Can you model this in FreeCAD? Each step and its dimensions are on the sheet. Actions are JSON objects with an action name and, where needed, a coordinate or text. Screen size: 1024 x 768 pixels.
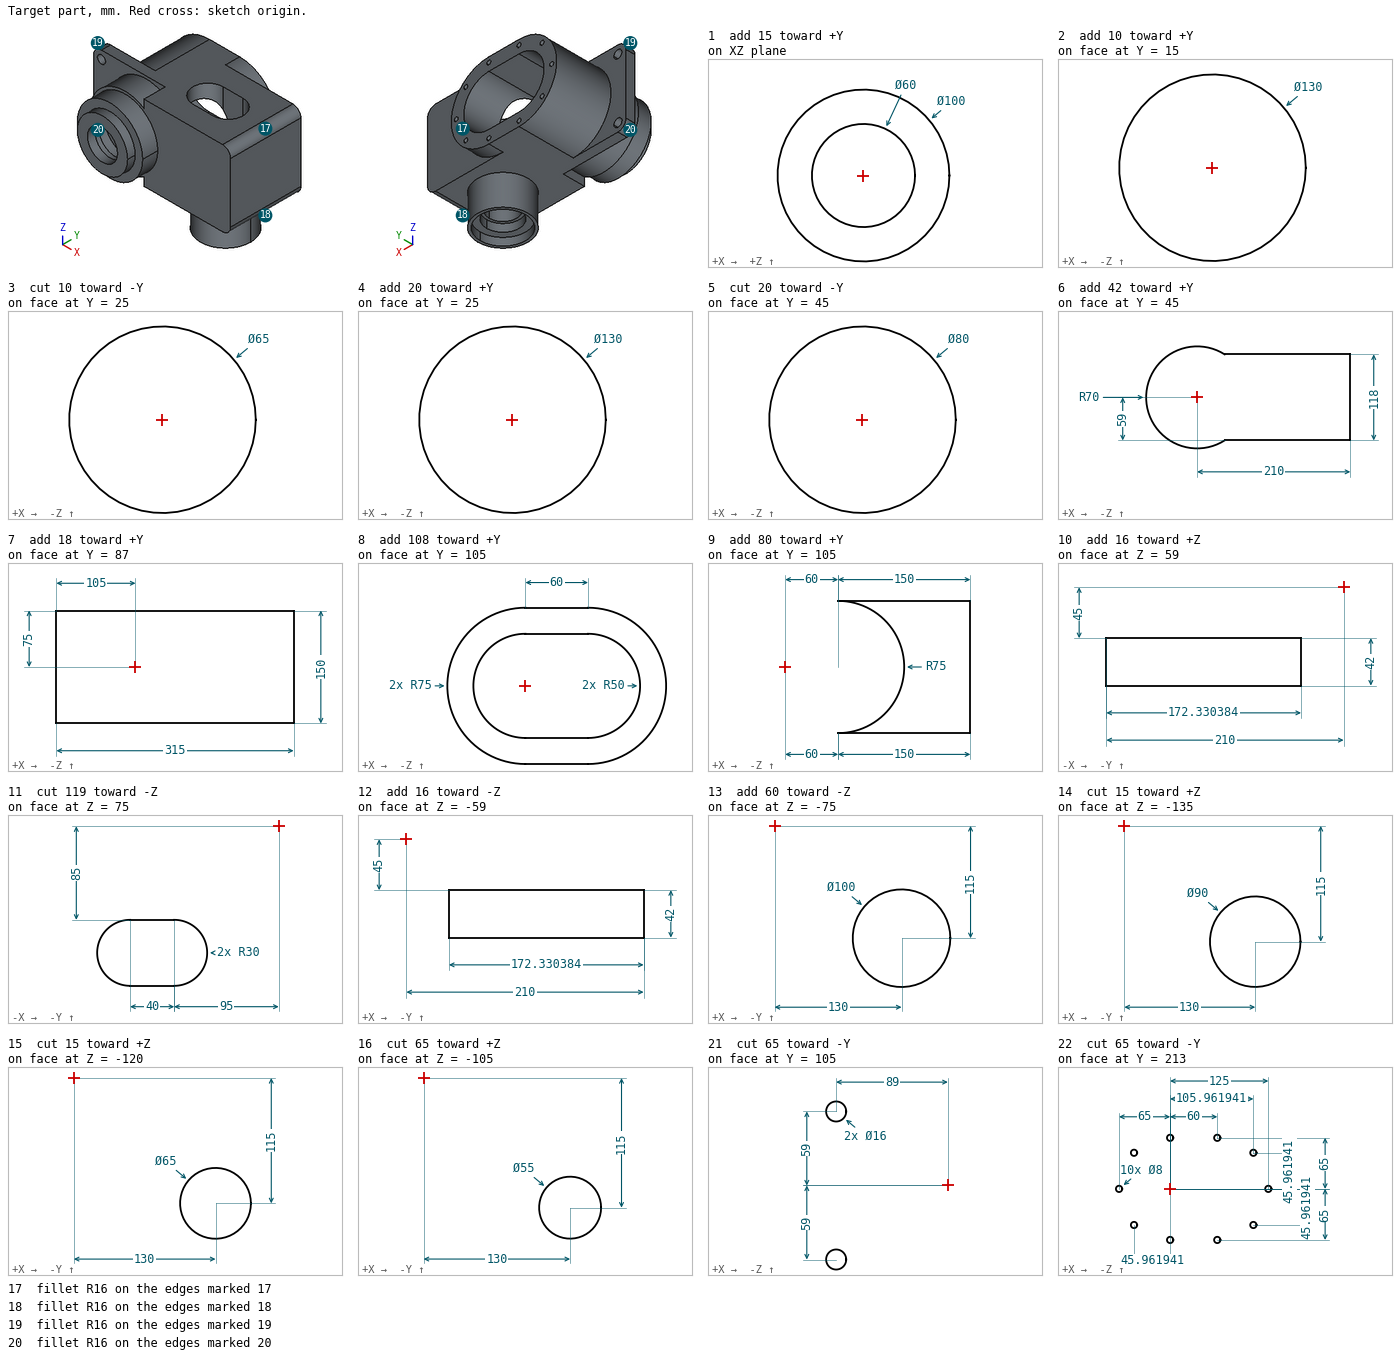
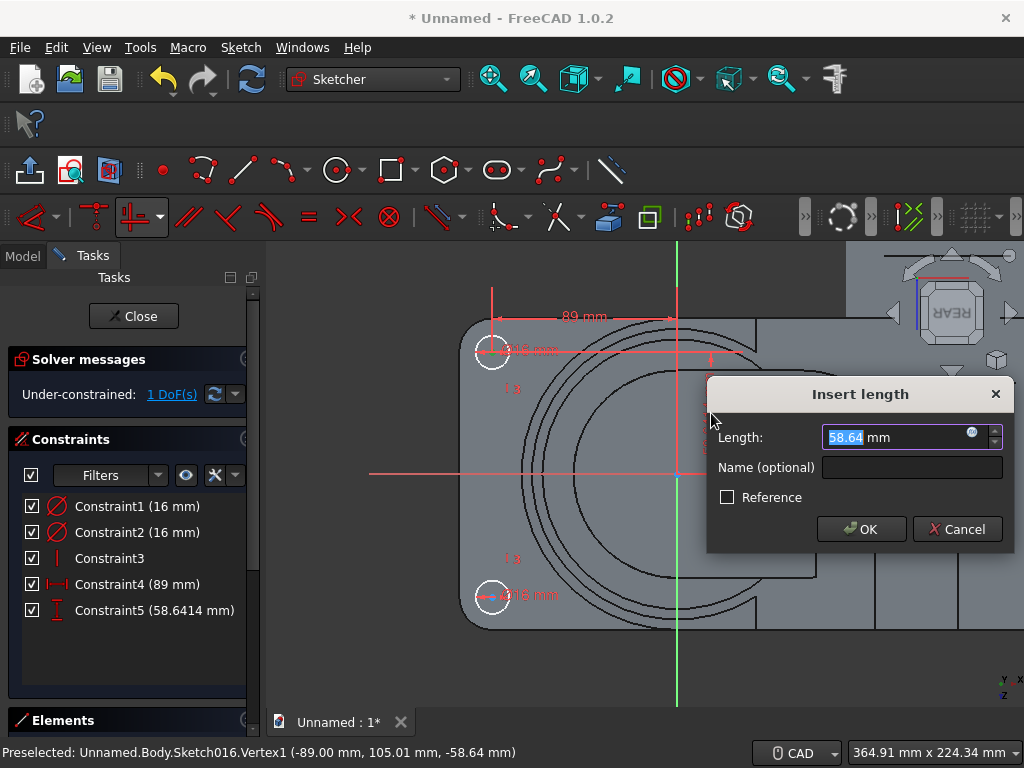
{"action": "type", "text": "59"}
{"action": "key", "text": "Return"}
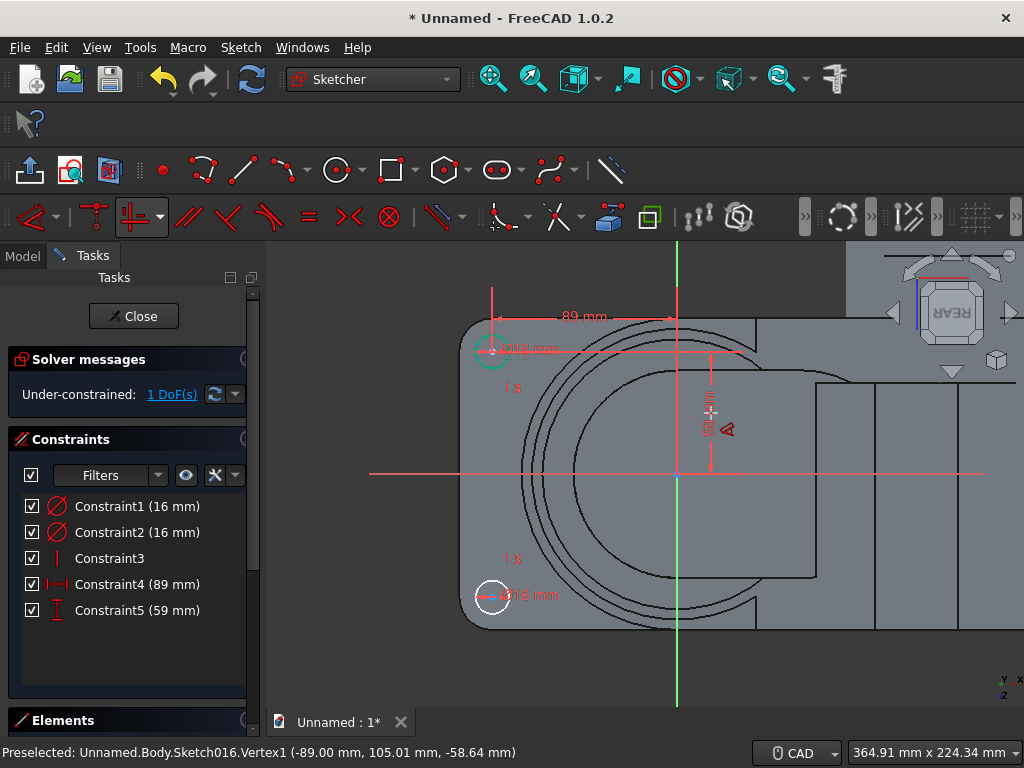
{"action": "left_click", "coordinate": [492, 597]}
{"action": "left_click", "coordinate": [711, 536]}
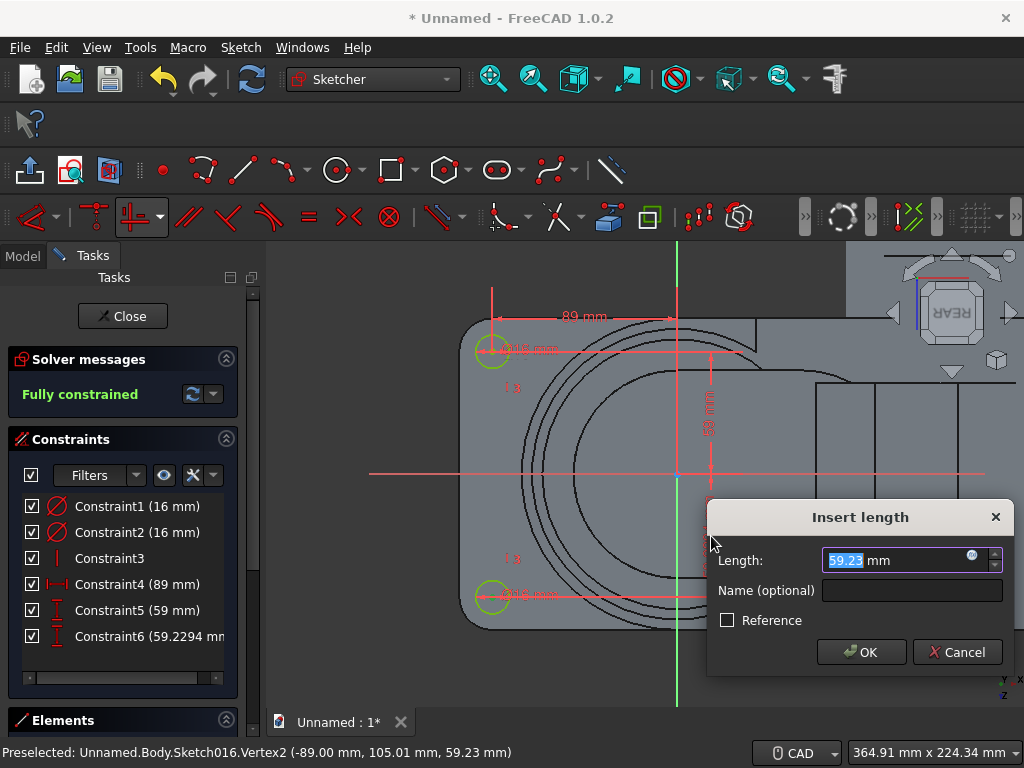
{"action": "type", "text": "59"}
{"action": "key", "text": "Return"}
{"action": "key", "text": "Escape"}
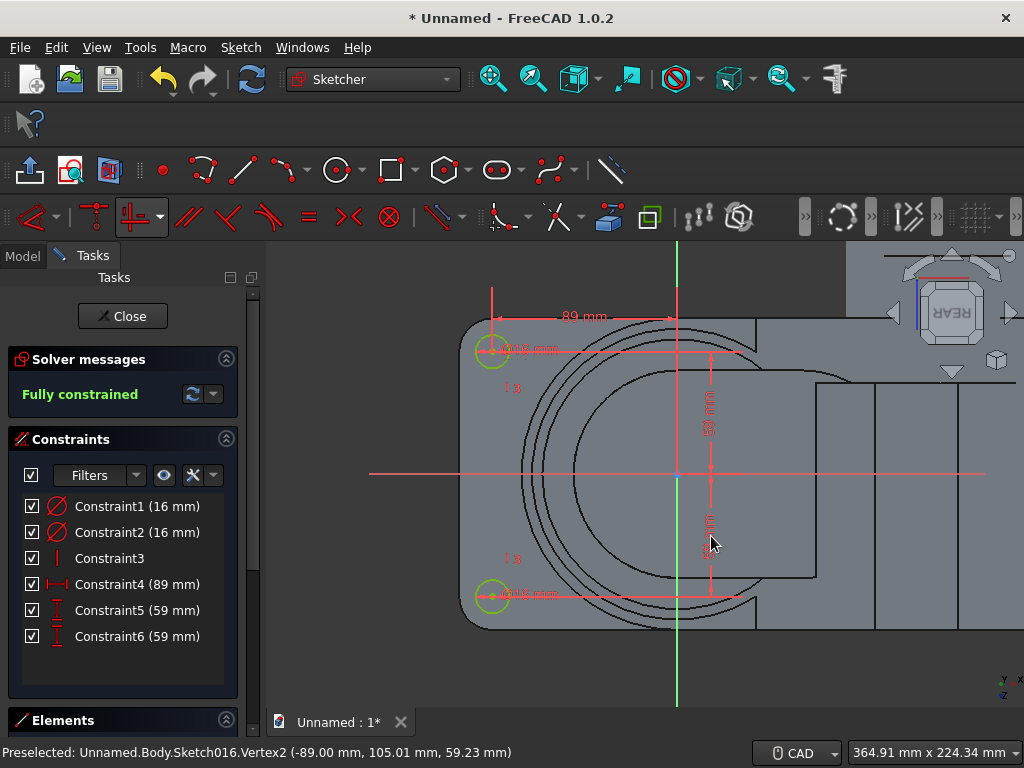
{"action": "left_click", "coordinate": [123, 316]}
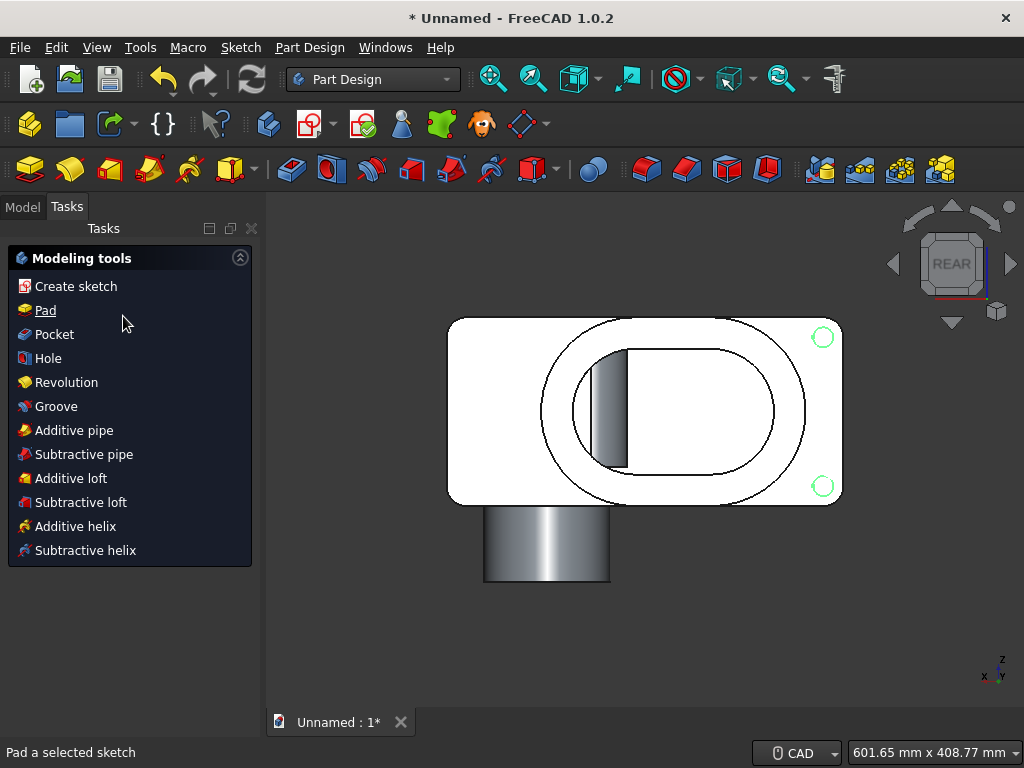
{"action": "left_click", "coordinate": [292, 170]}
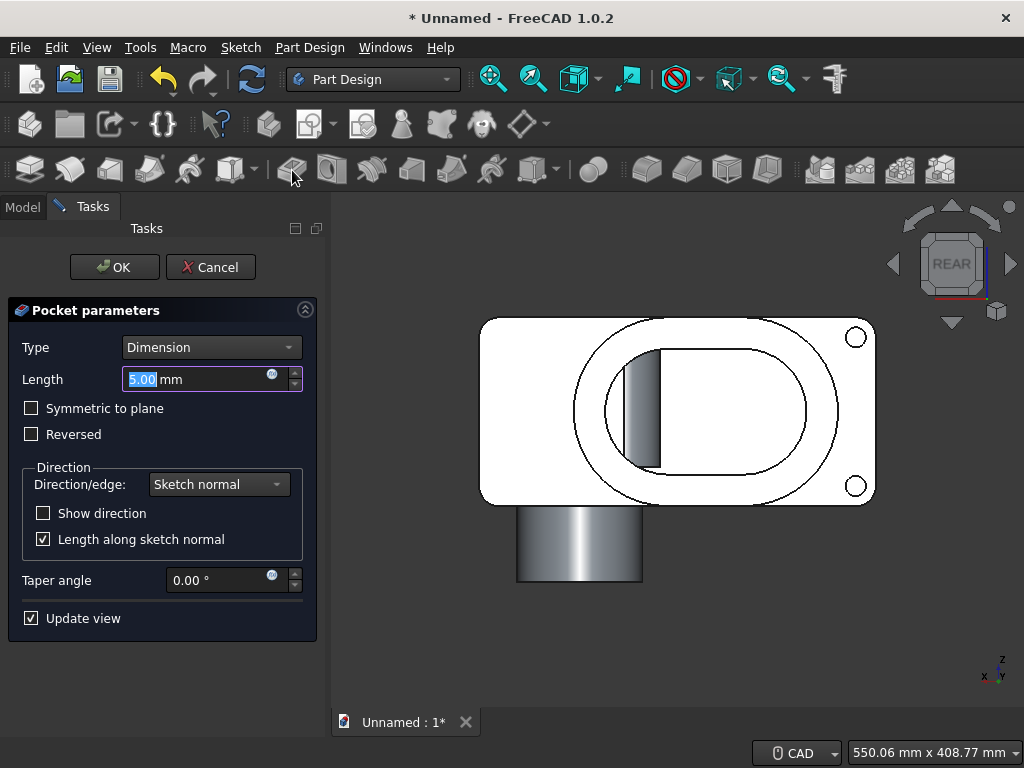
{"action": "type", "text": "65"}
{"action": "key", "text": "Tab"}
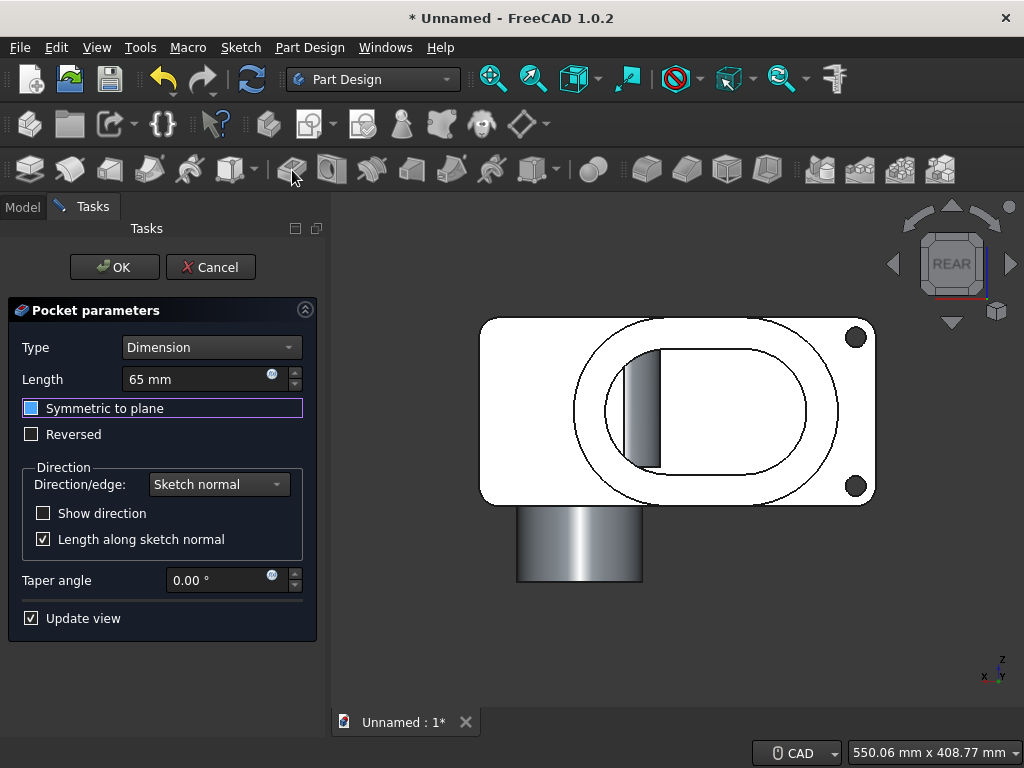
{"action": "left_click", "coordinate": [115, 267]}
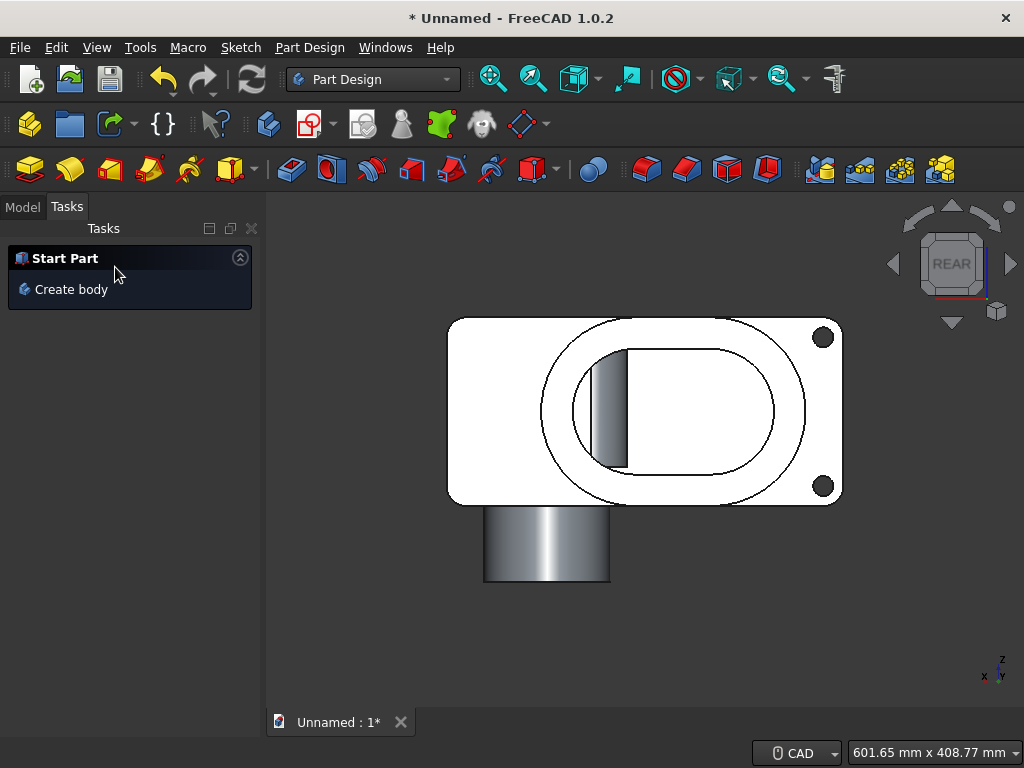
{"action": "left_click", "coordinate": [560, 438]}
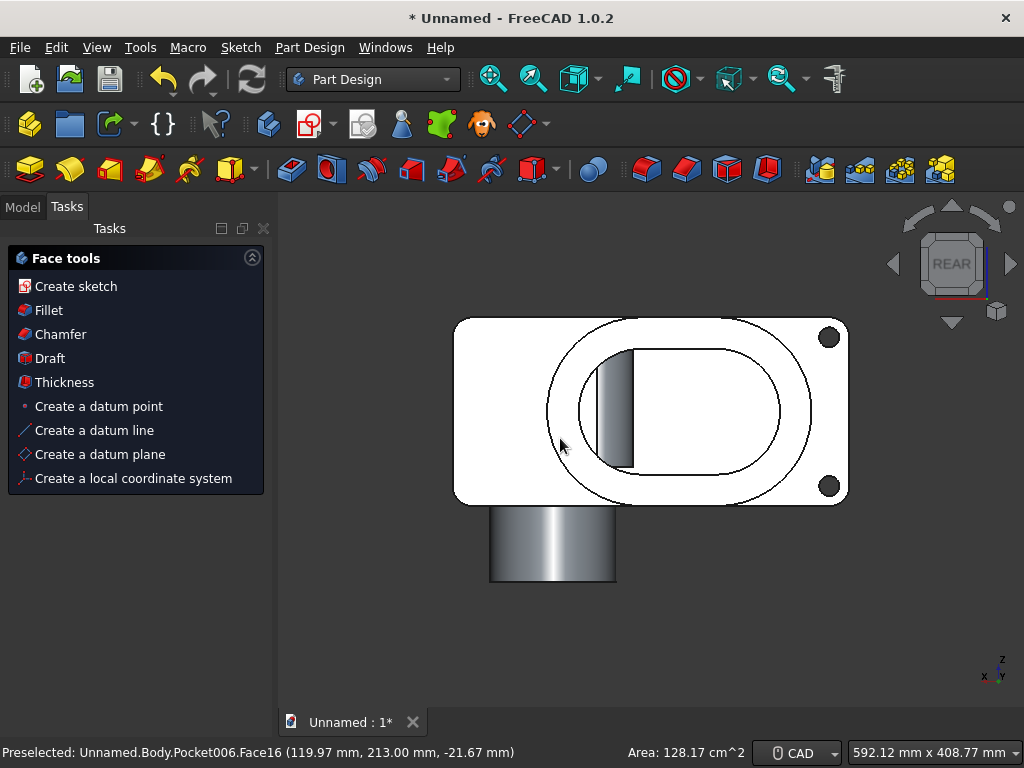
{"action": "left_click", "coordinate": [310, 124]}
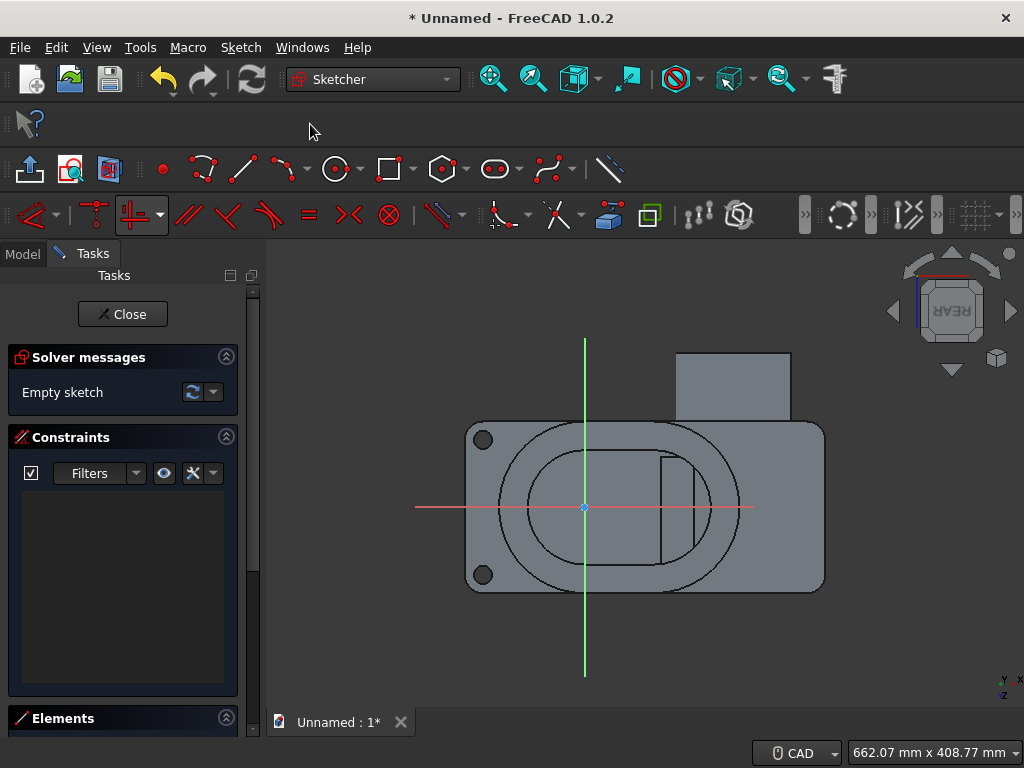
{"action": "scroll", "coordinate": [671, 549], "scroll_direction": "up", "scroll_amount": 3}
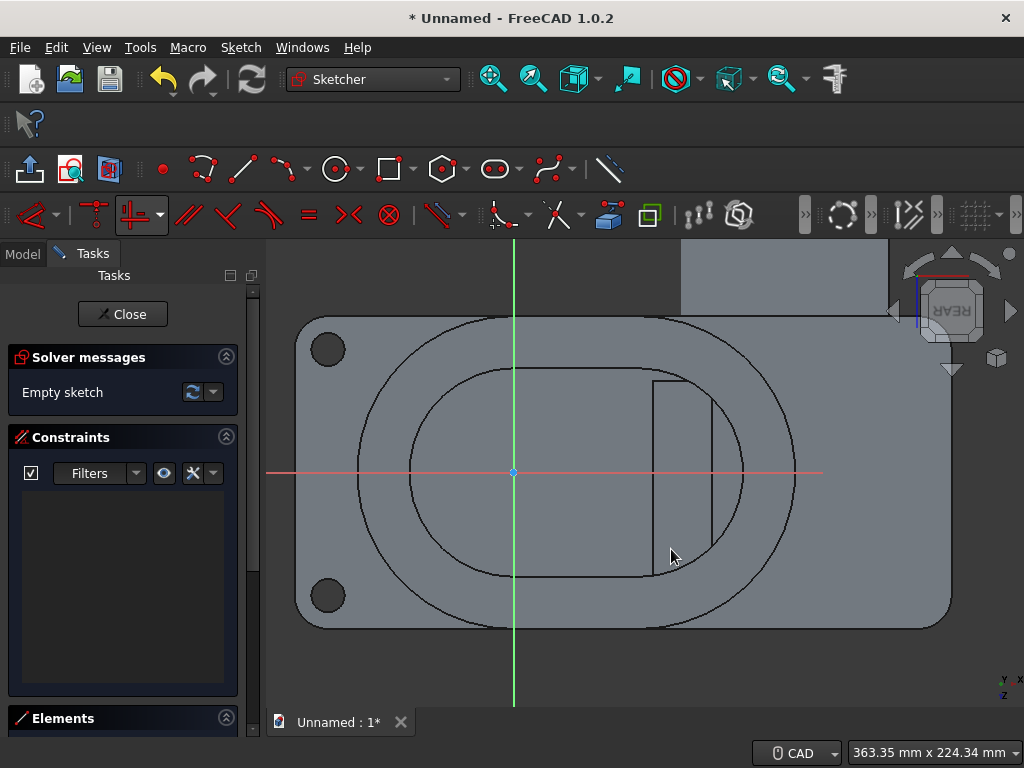
{"action": "left_click", "coordinate": [336, 170]}